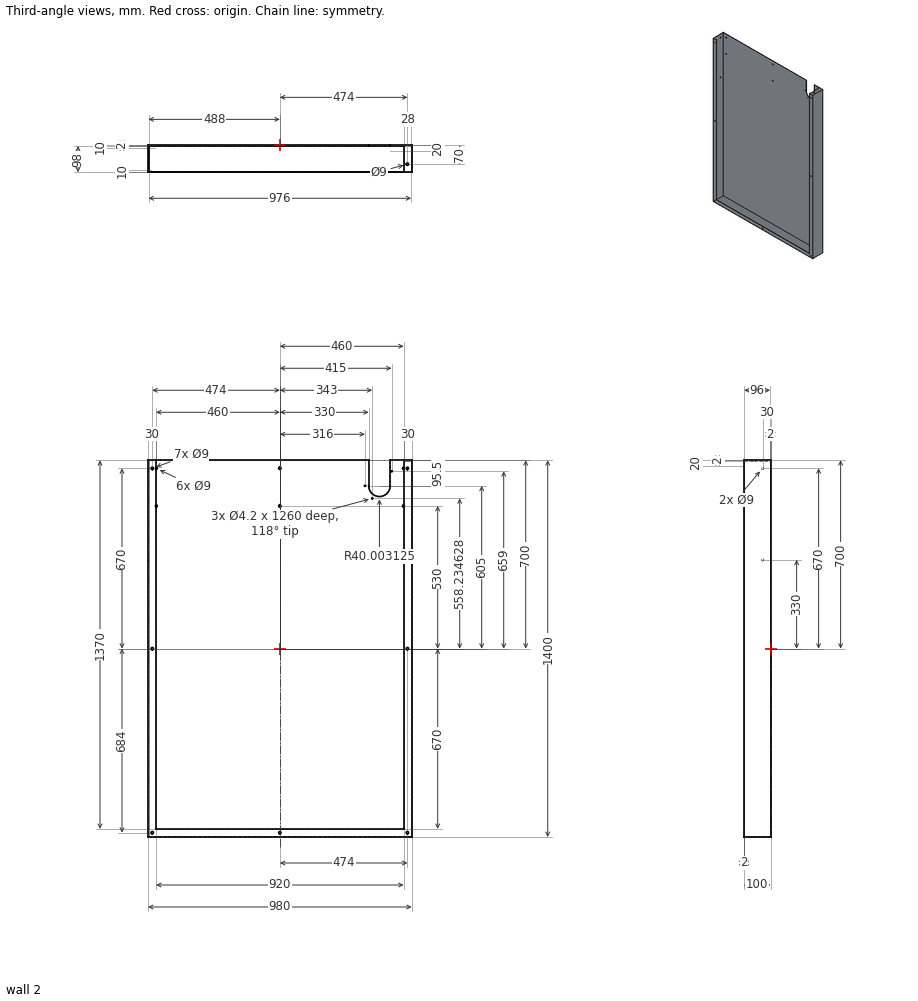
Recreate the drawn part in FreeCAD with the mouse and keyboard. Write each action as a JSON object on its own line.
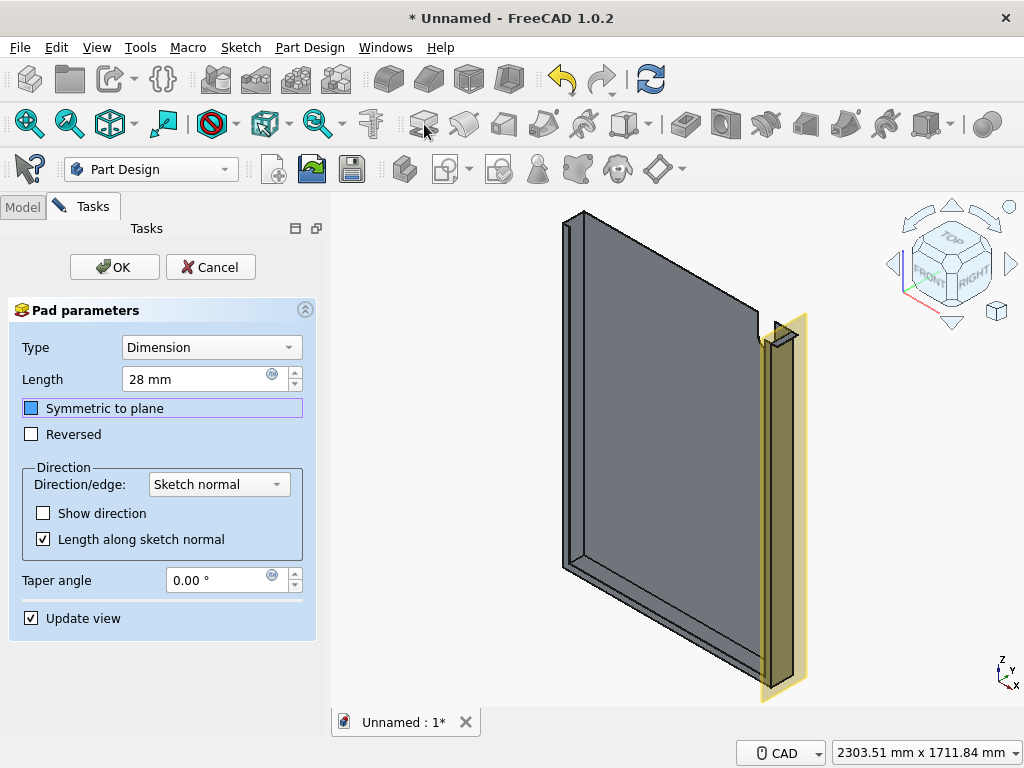
{"action": "left_click", "coordinate": [30, 434]}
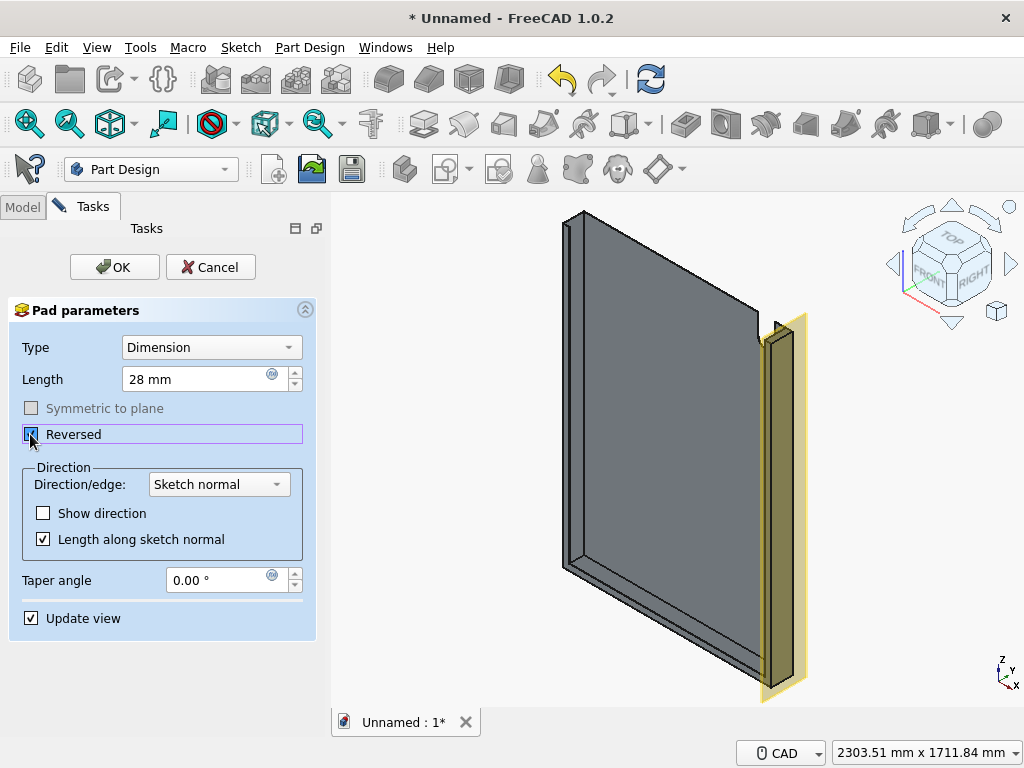
{"action": "left_click", "coordinate": [115, 267]}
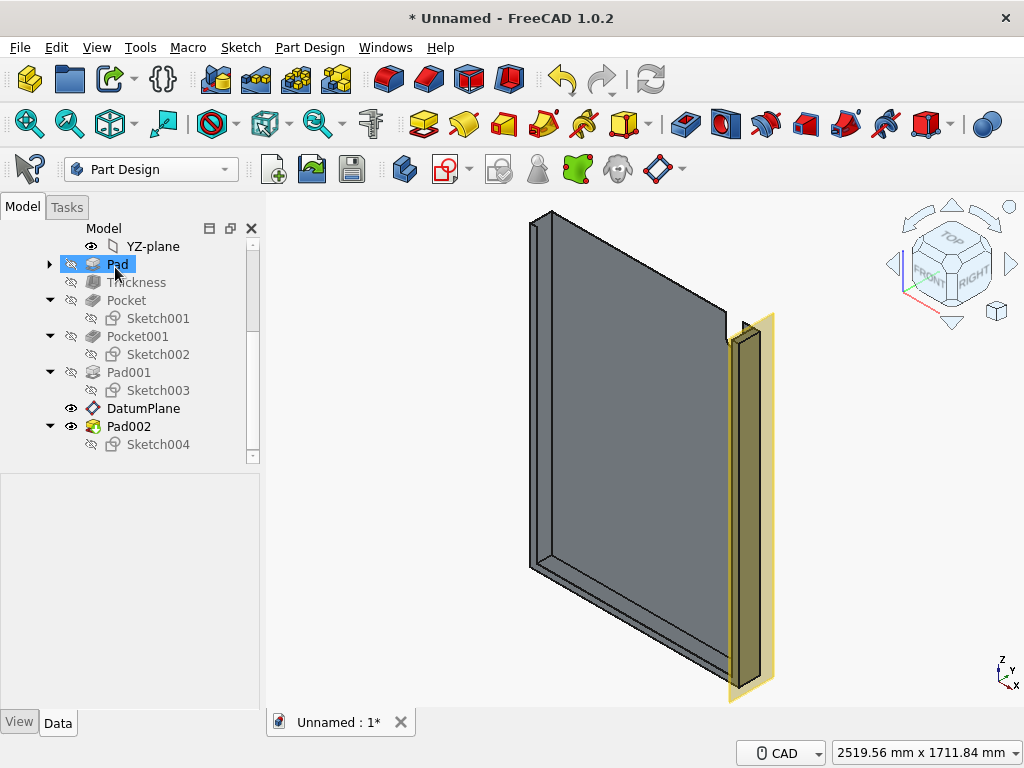
{"action": "left_click", "coordinate": [116, 408]}
{"action": "key", "text": "space"}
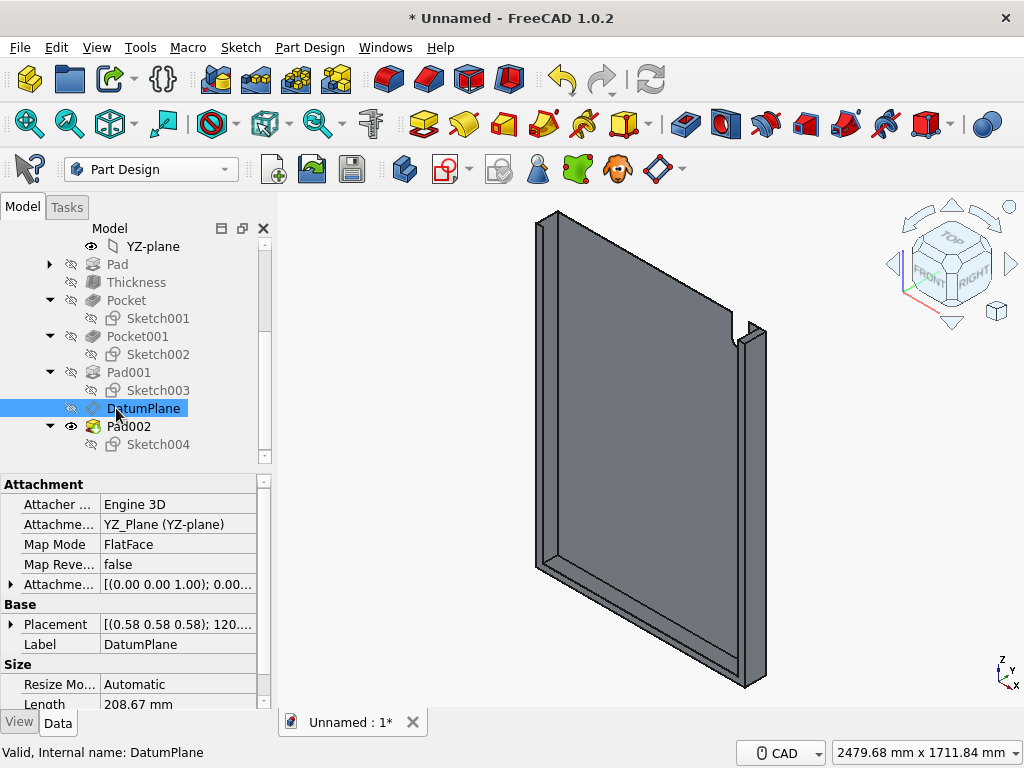
{"action": "scroll", "coordinate": [743, 568], "scroll_direction": "up", "scroll_amount": 7}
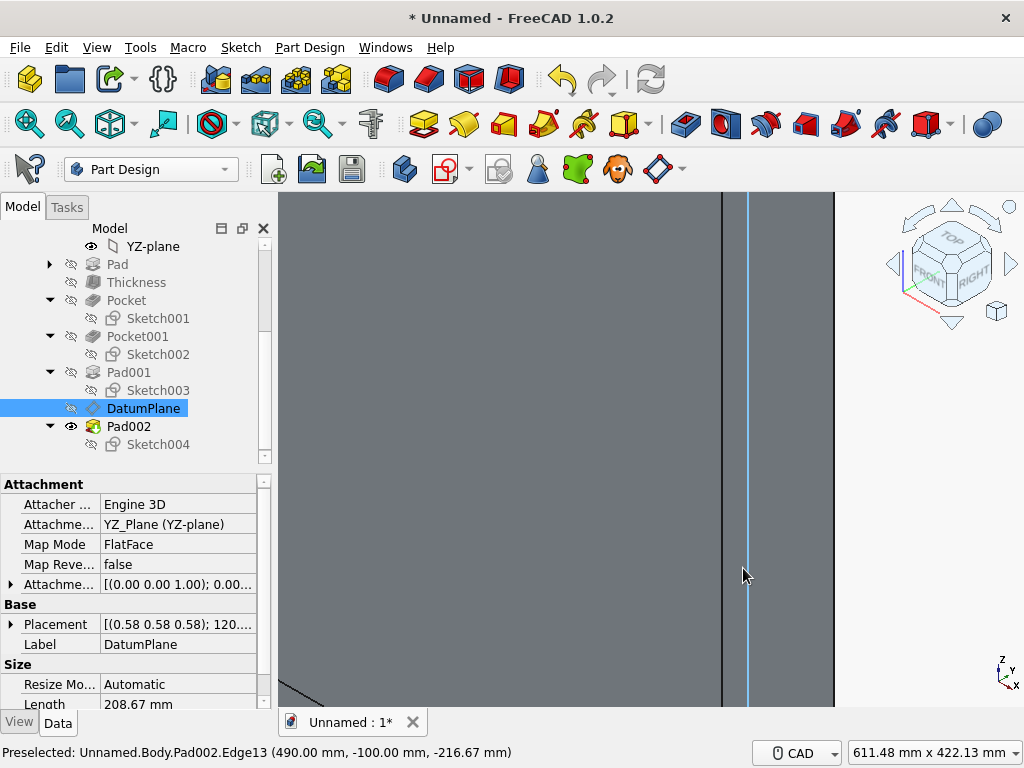
{"action": "left_click", "coordinate": [740, 570]}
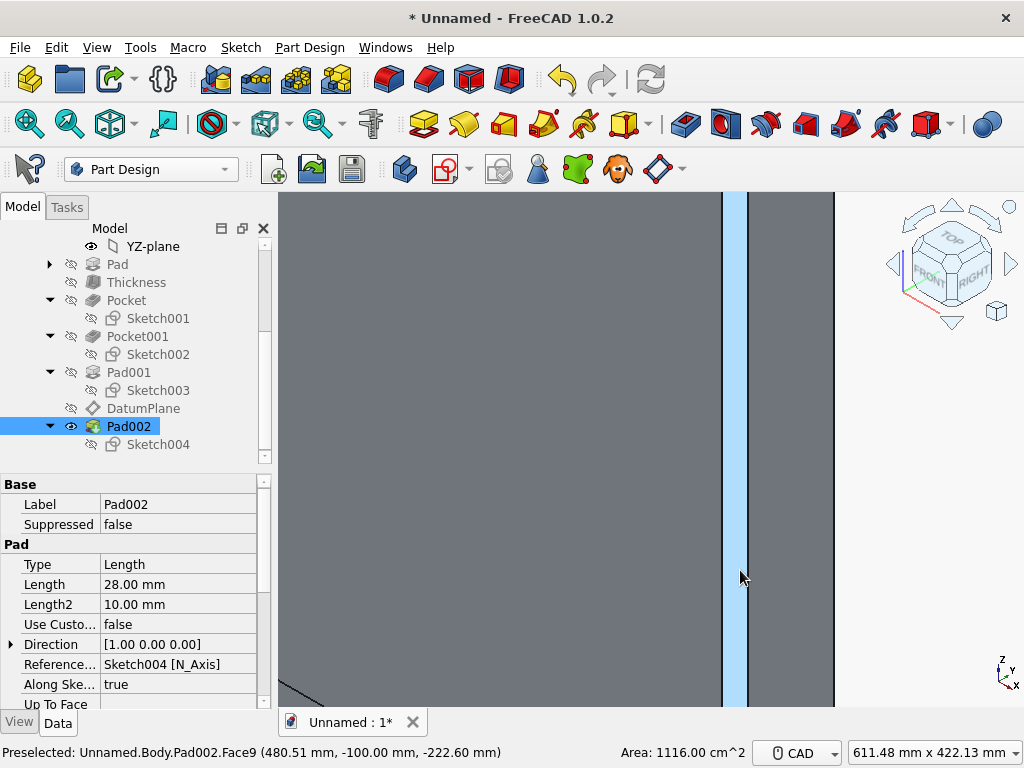
{"action": "left_click", "coordinate": [446, 170]}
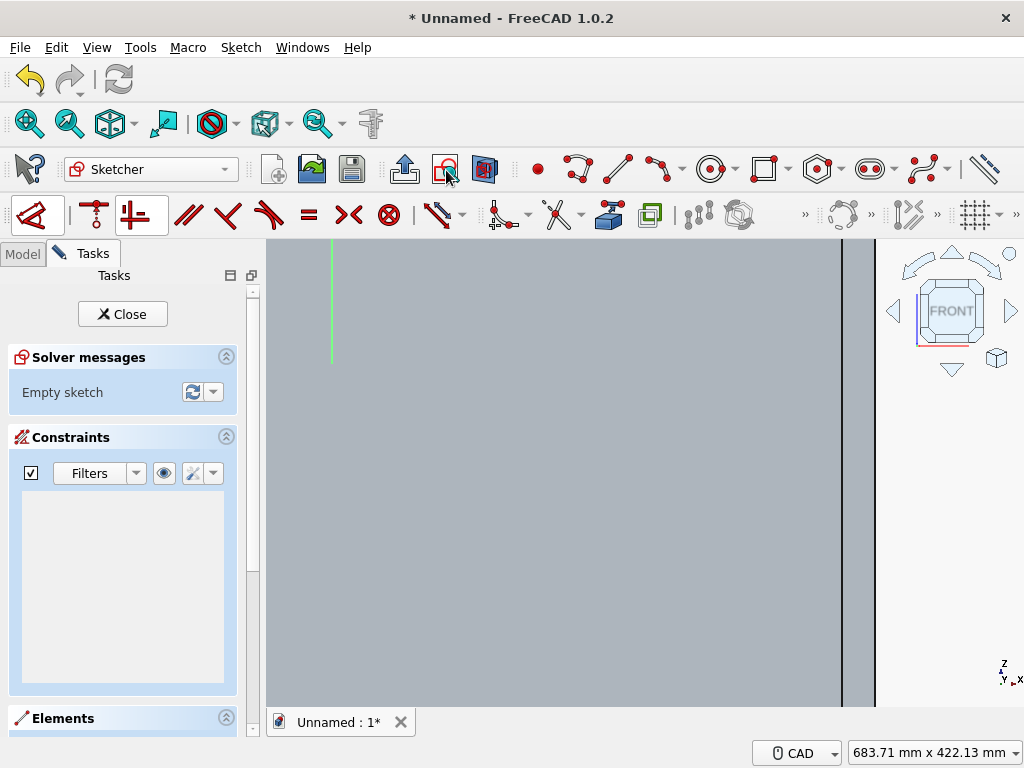
{"action": "scroll", "coordinate": [638, 540], "scroll_direction": "down", "scroll_amount": 8}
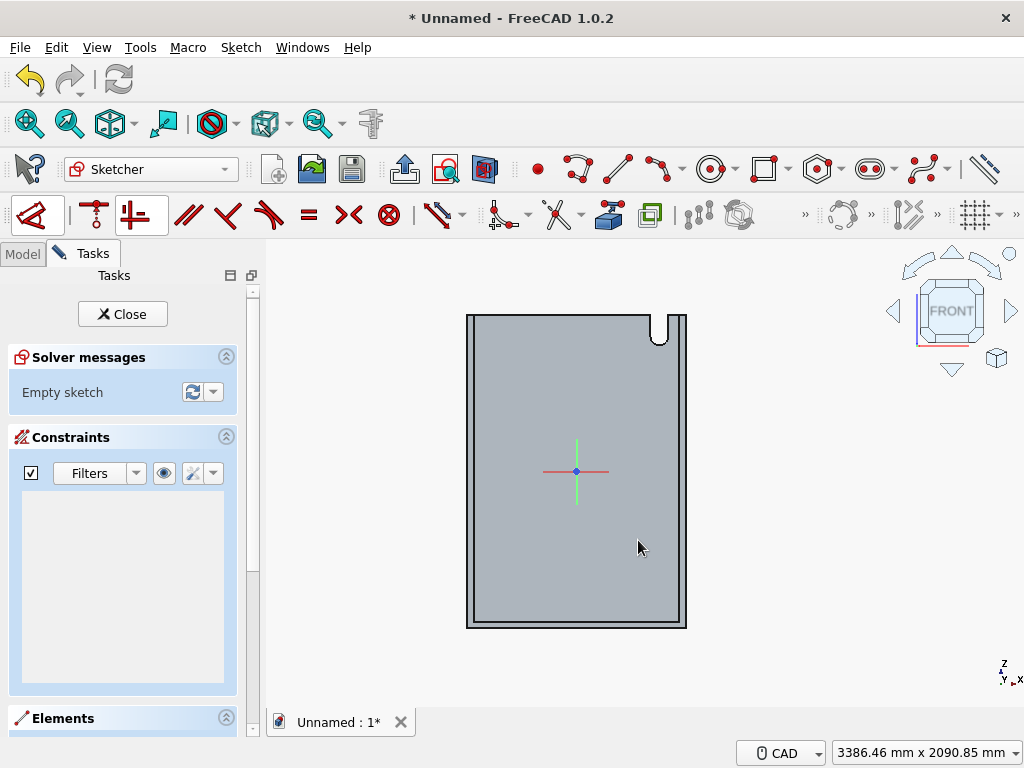
{"action": "left_click", "coordinate": [712, 170]}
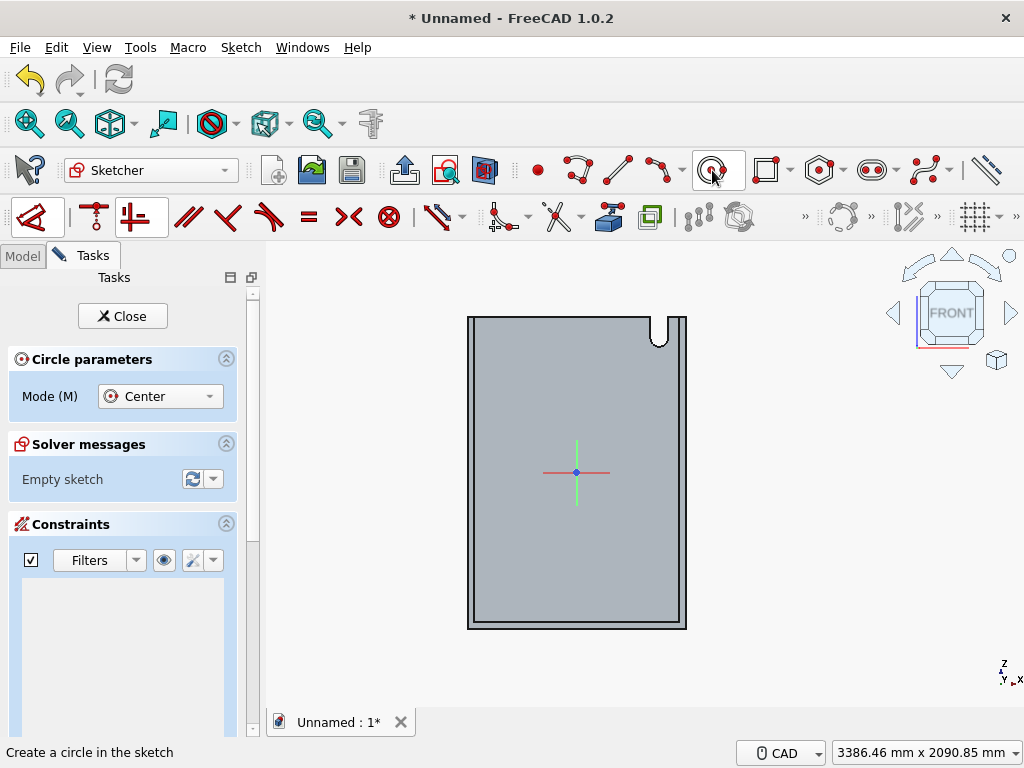
{"action": "scroll", "coordinate": [471, 323], "scroll_direction": "up", "scroll_amount": 16}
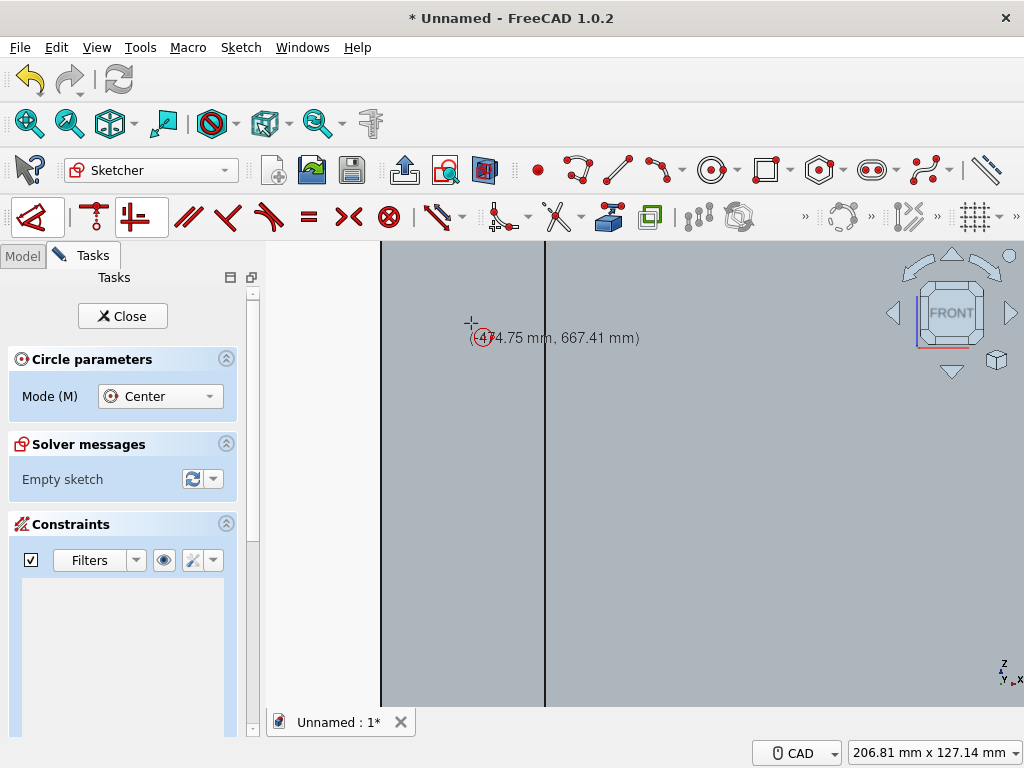
{"action": "scroll", "coordinate": [471, 323], "scroll_direction": "down", "scroll_amount": 16}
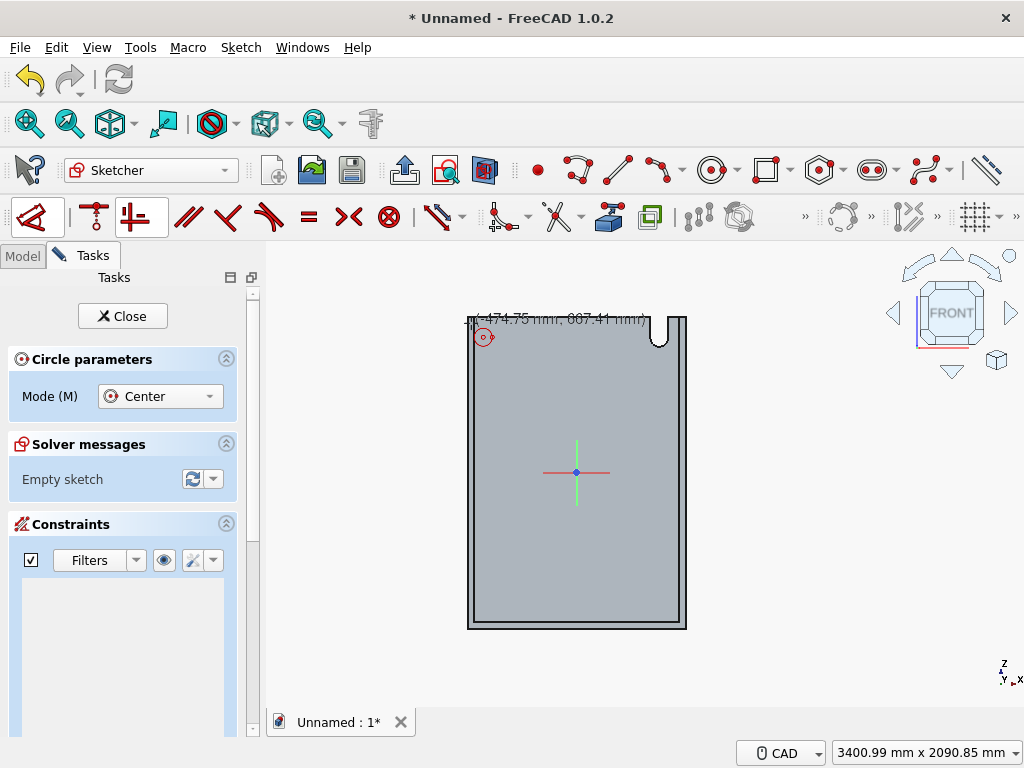
{"action": "left_click", "coordinate": [471, 323]}
{"action": "mouse_move", "coordinate": [472, 323]}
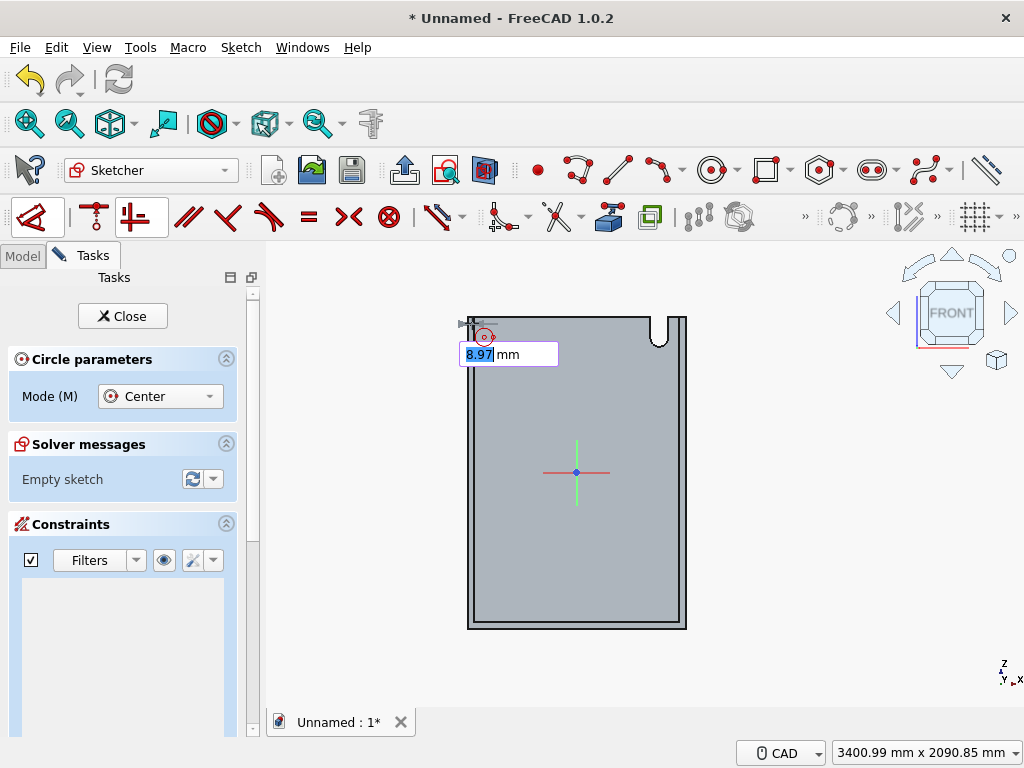
{"action": "type", "text": "9"}
{"action": "key", "text": "Return"}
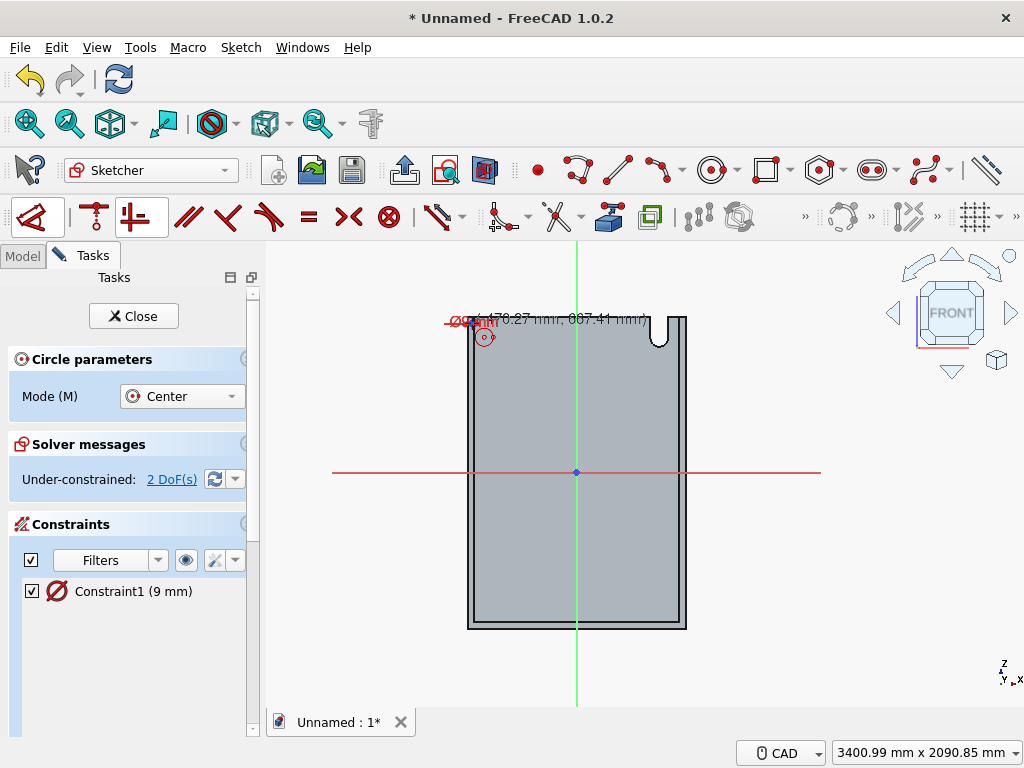
{"action": "scroll", "coordinate": [471, 473], "scroll_direction": "up", "scroll_amount": 16}